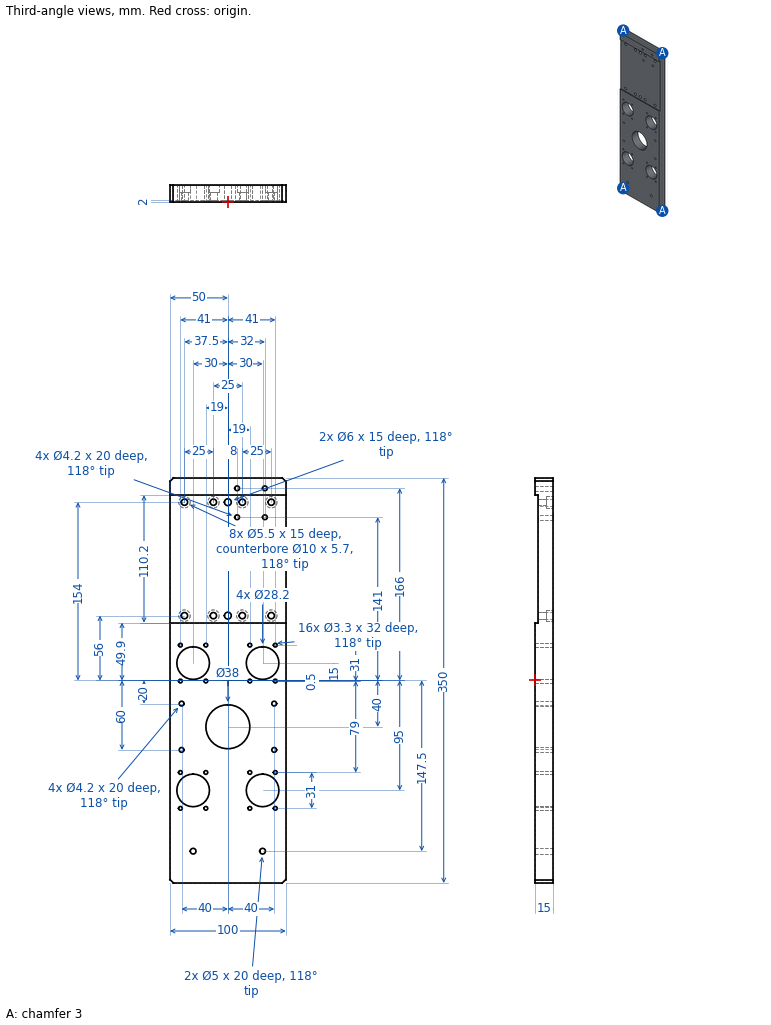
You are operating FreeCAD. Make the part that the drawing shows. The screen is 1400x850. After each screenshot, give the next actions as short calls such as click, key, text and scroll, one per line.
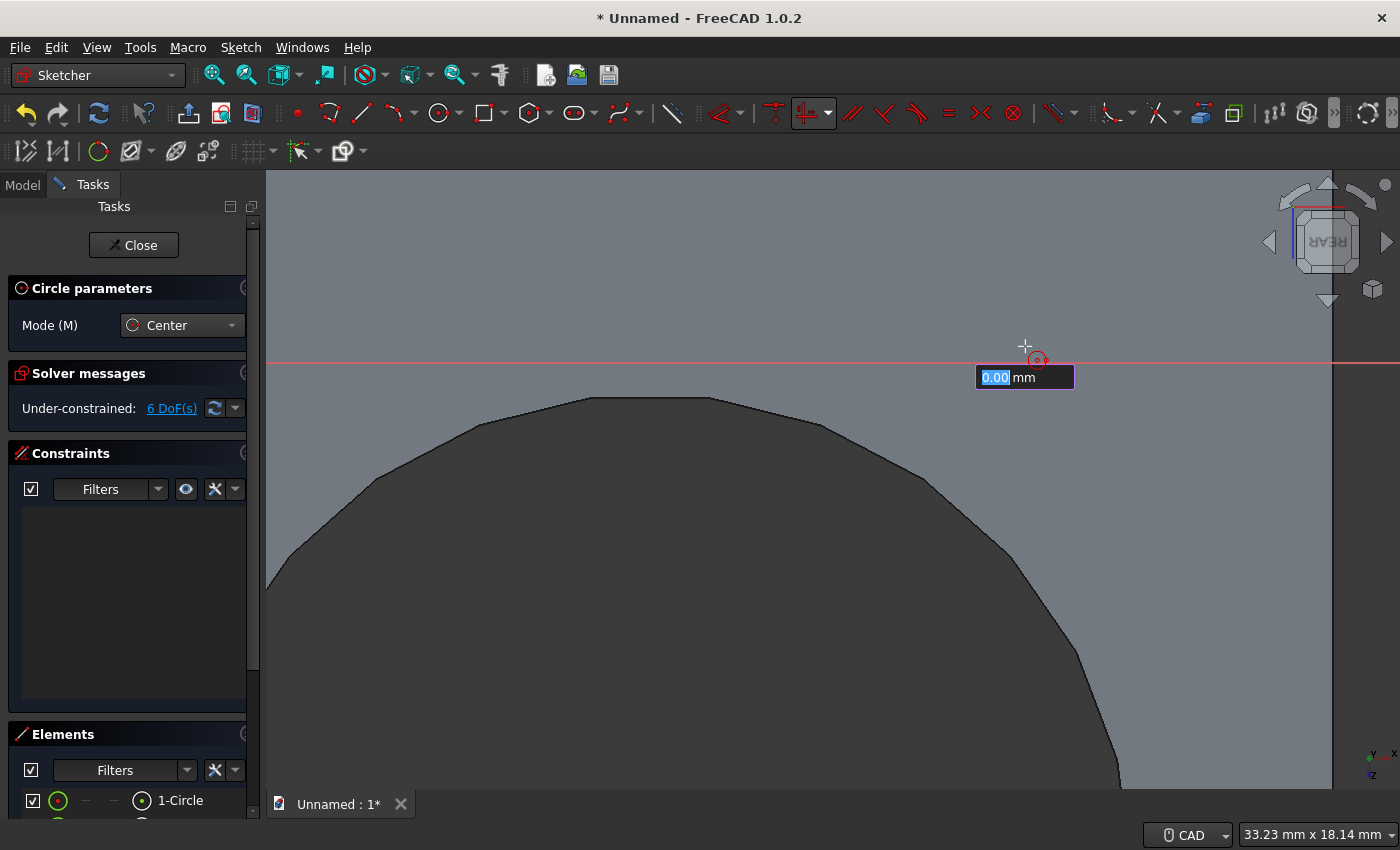
scroll(856, 598, down, 13)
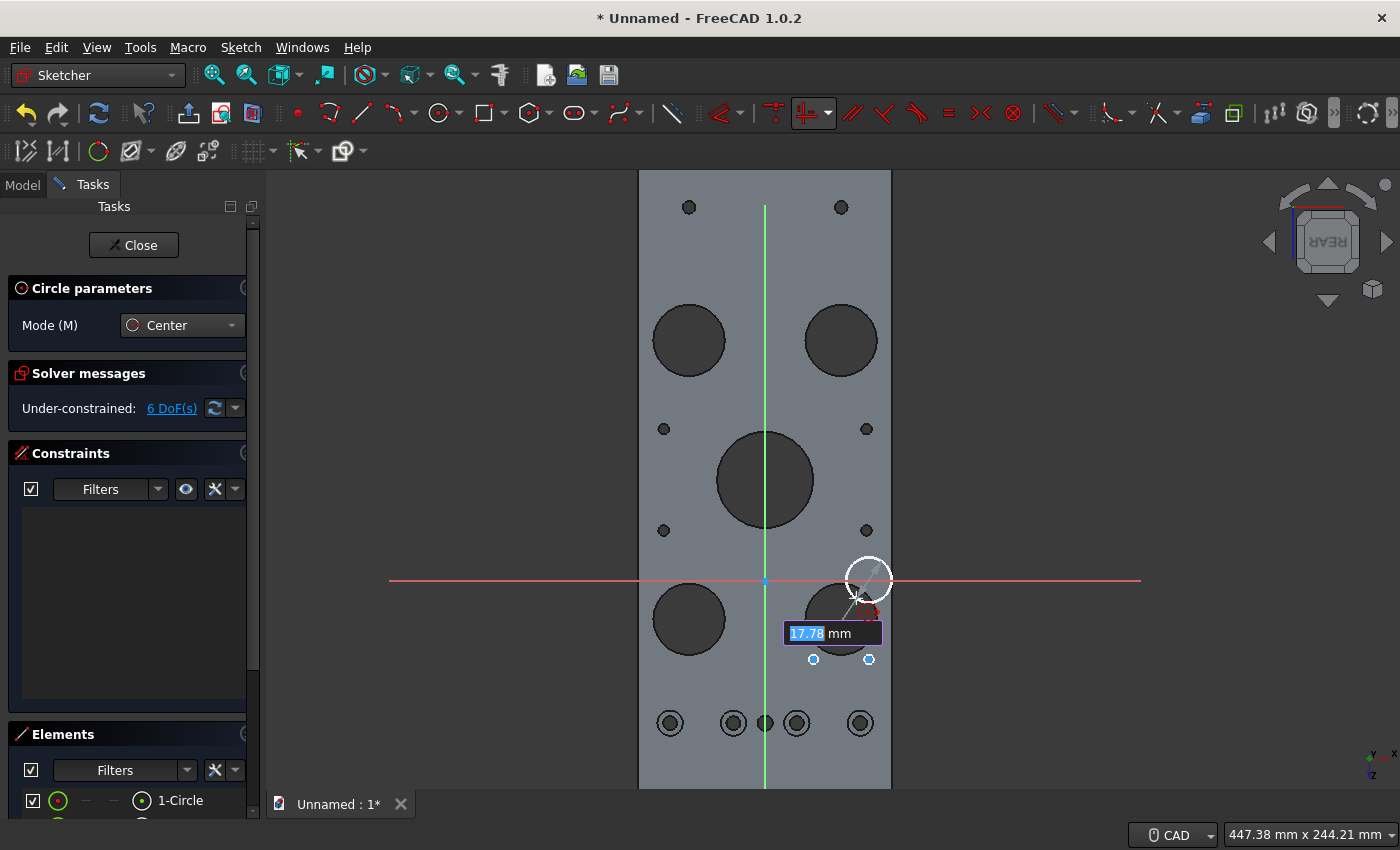
scroll(872, 577, up, 7)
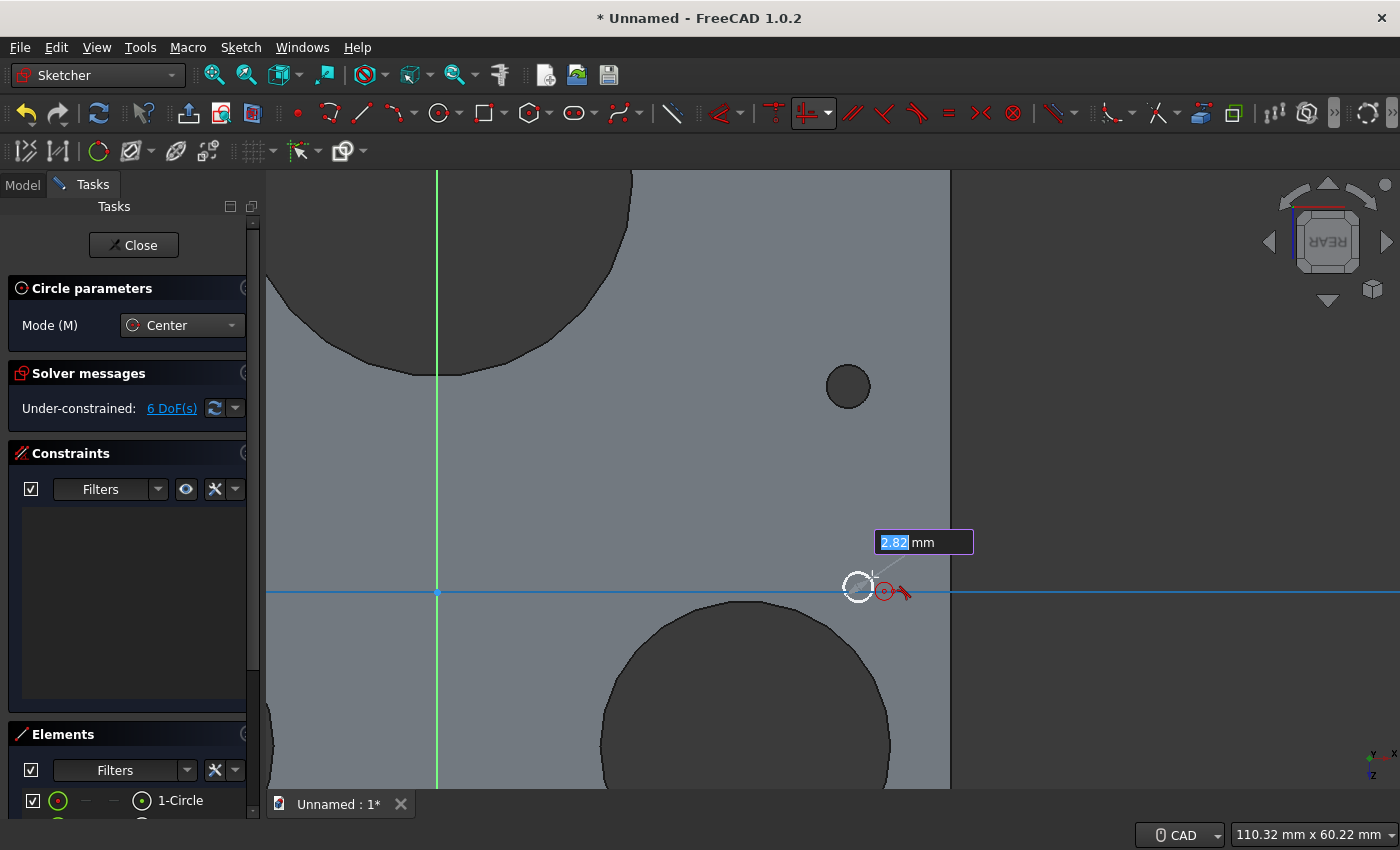
click(870, 575)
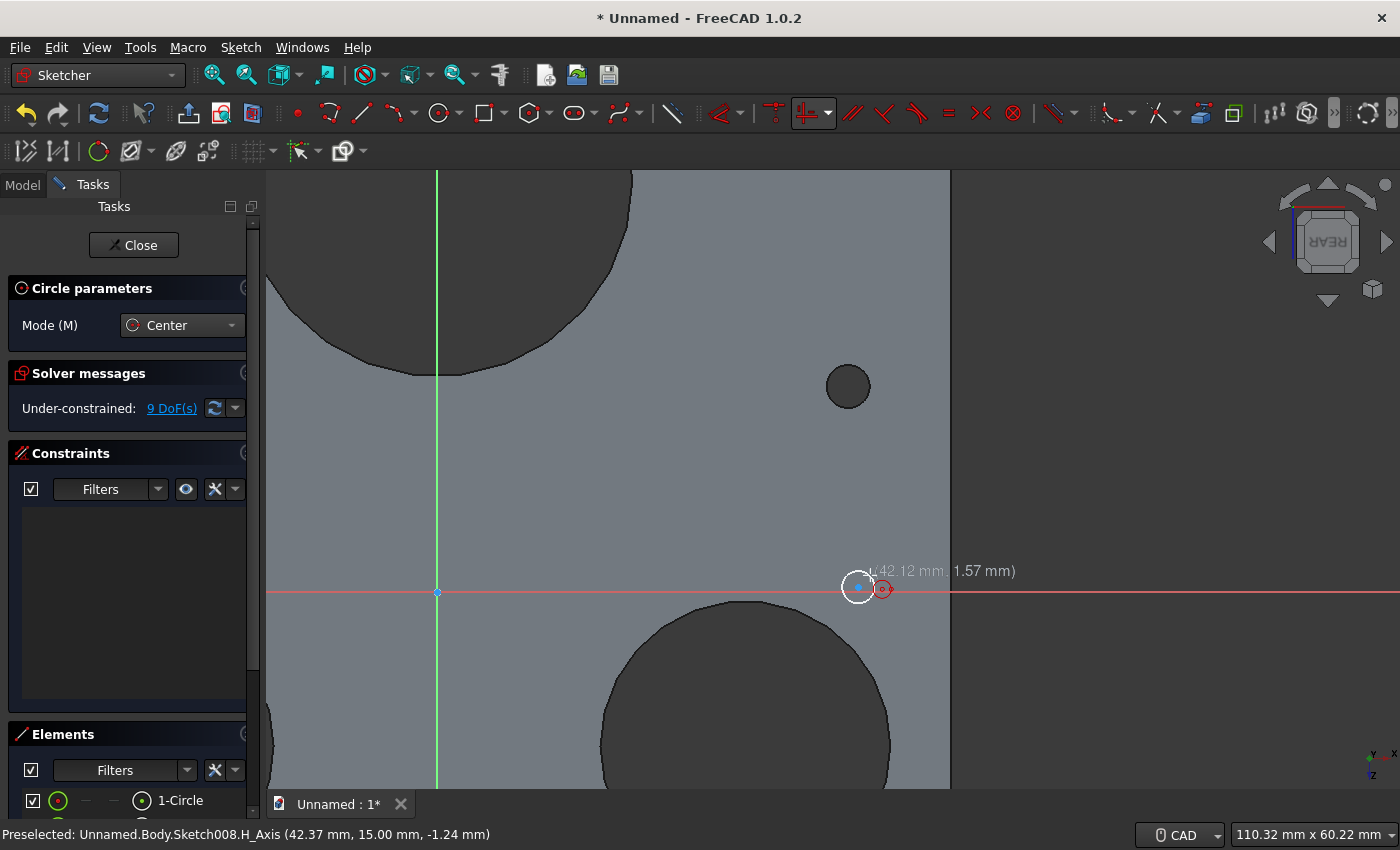
scroll(632, 587, up, 6)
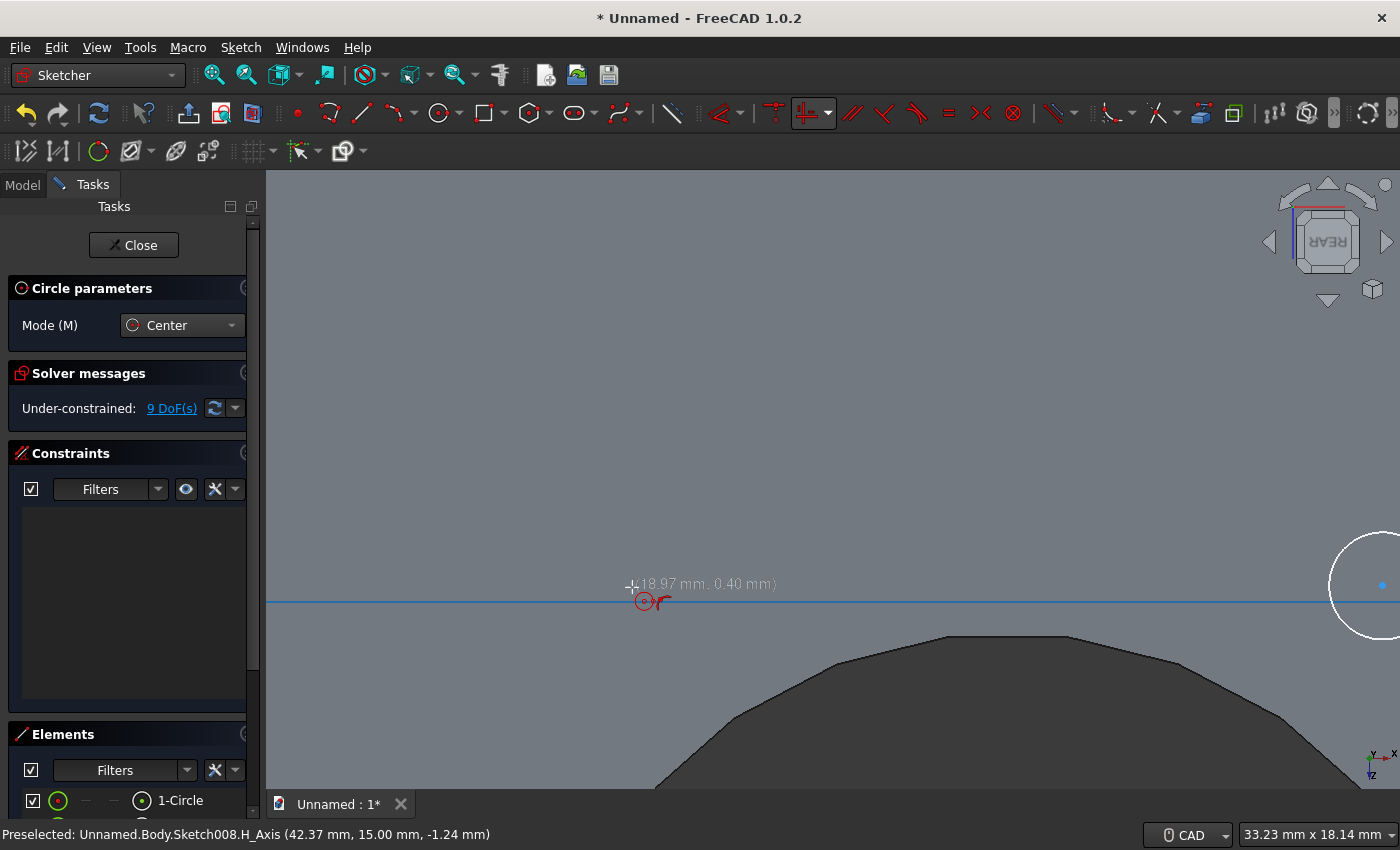
click(632, 585)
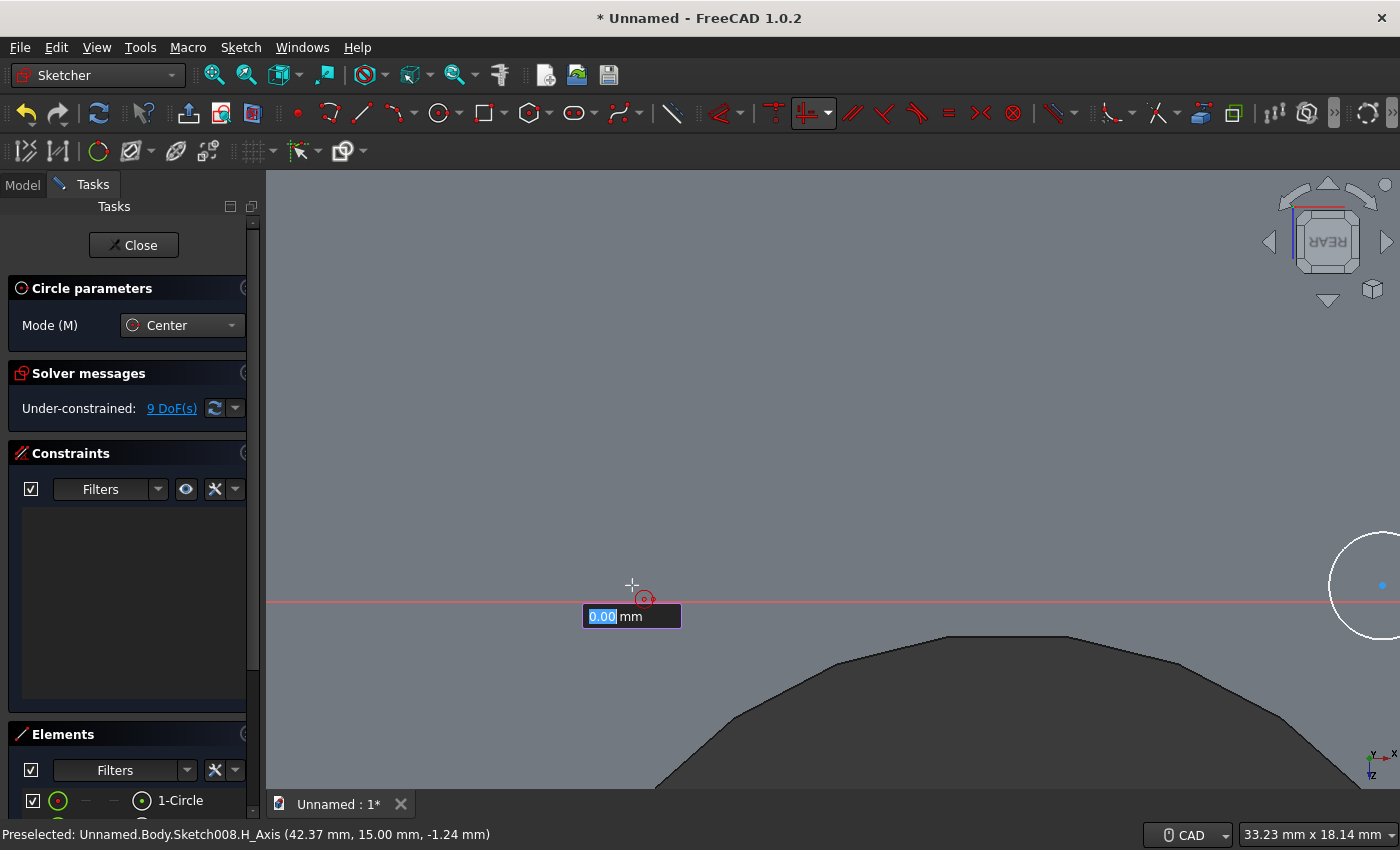
scroll(827, 579, down, 13)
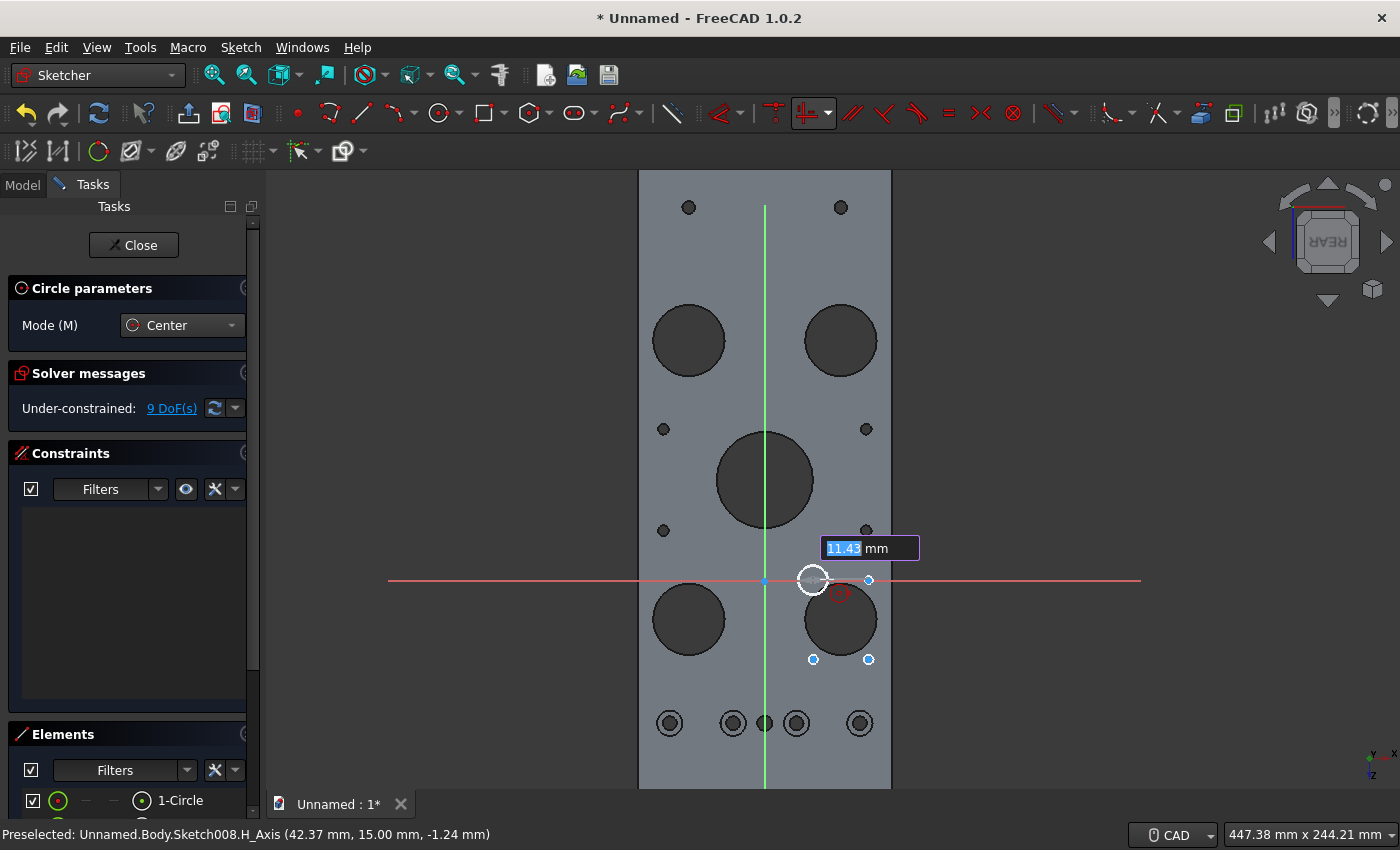
scroll(816, 577, up, 7)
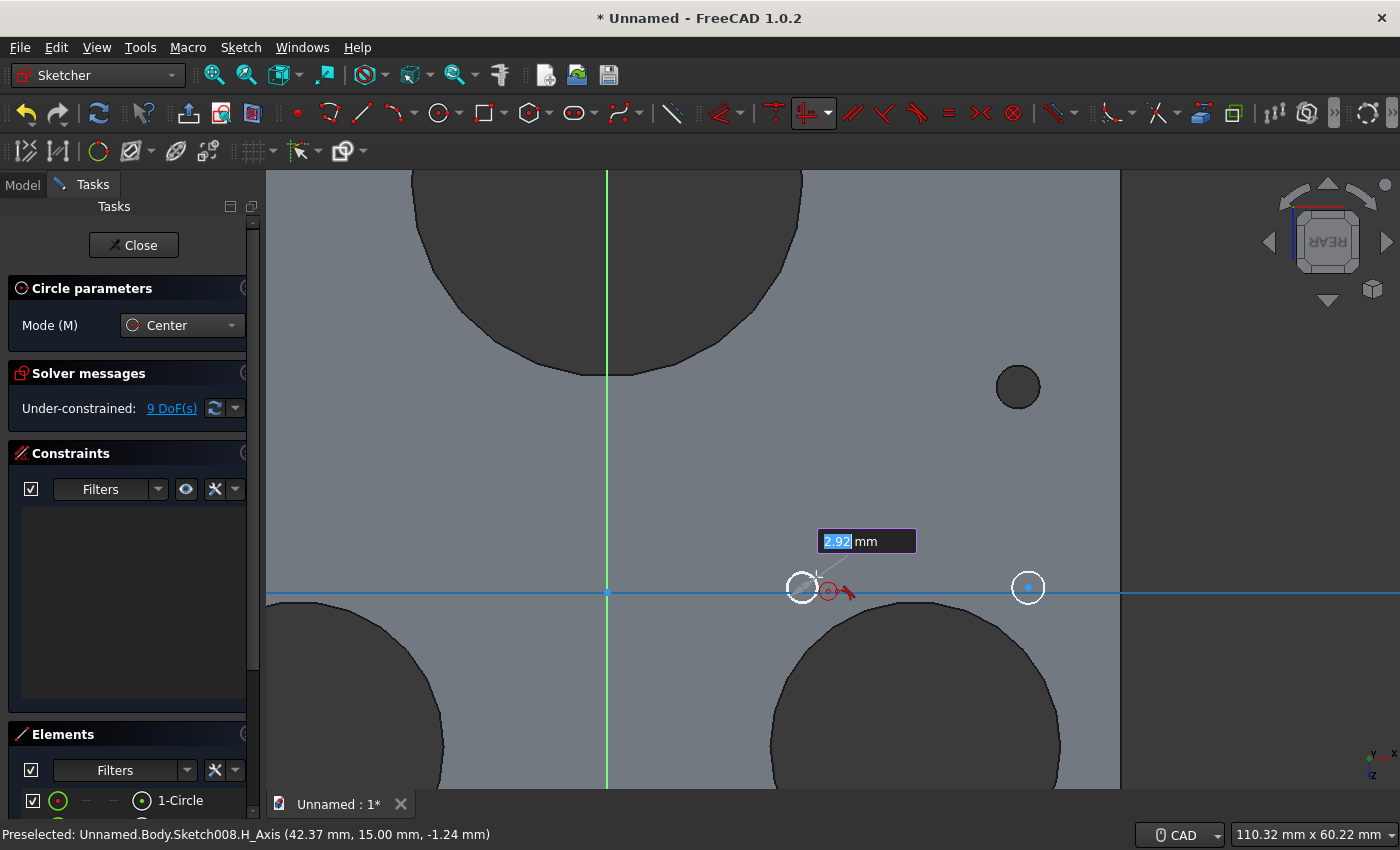
click(814, 575)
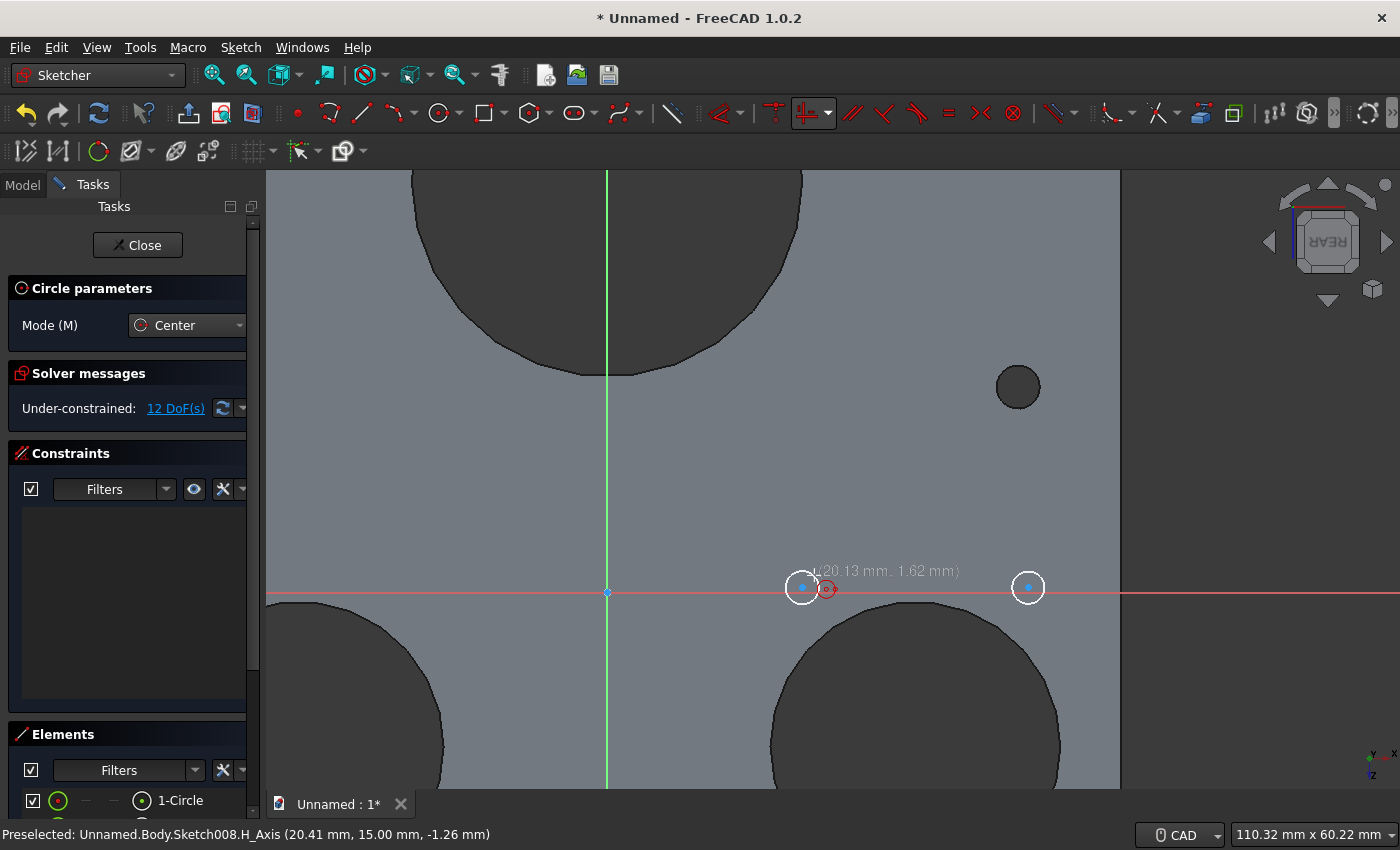
scroll(816, 577, down, 7)